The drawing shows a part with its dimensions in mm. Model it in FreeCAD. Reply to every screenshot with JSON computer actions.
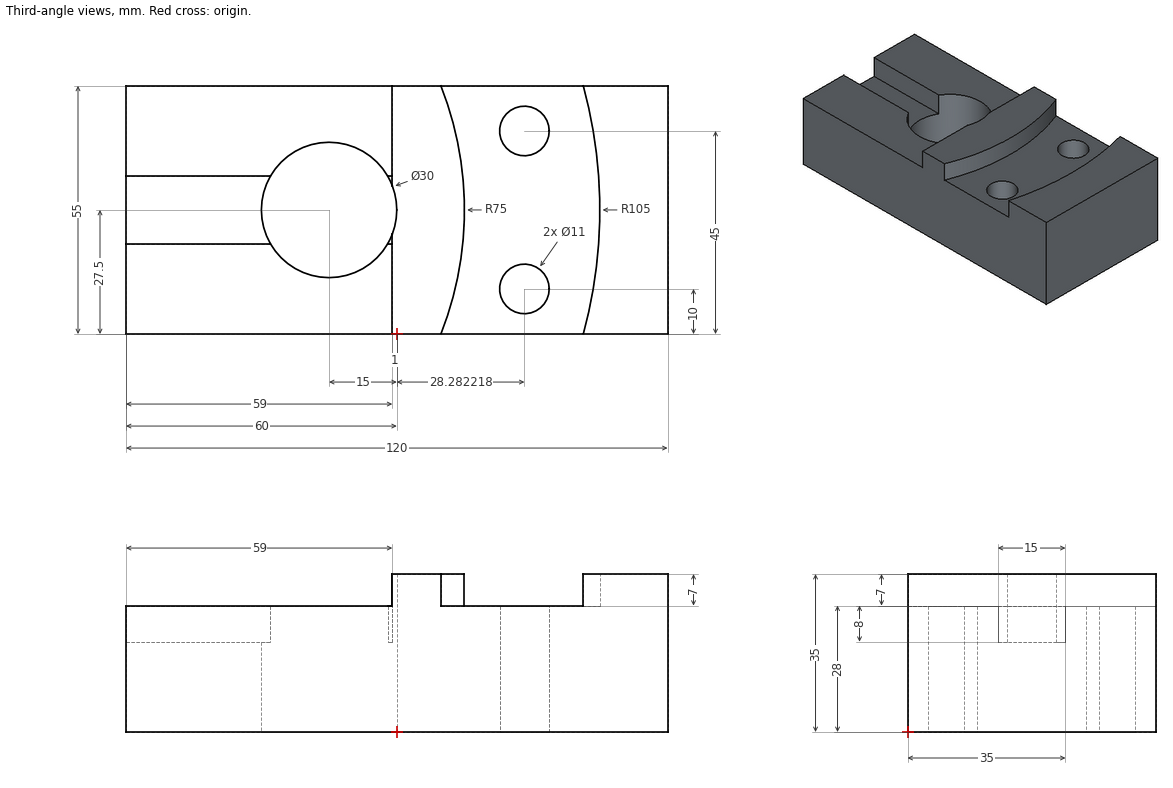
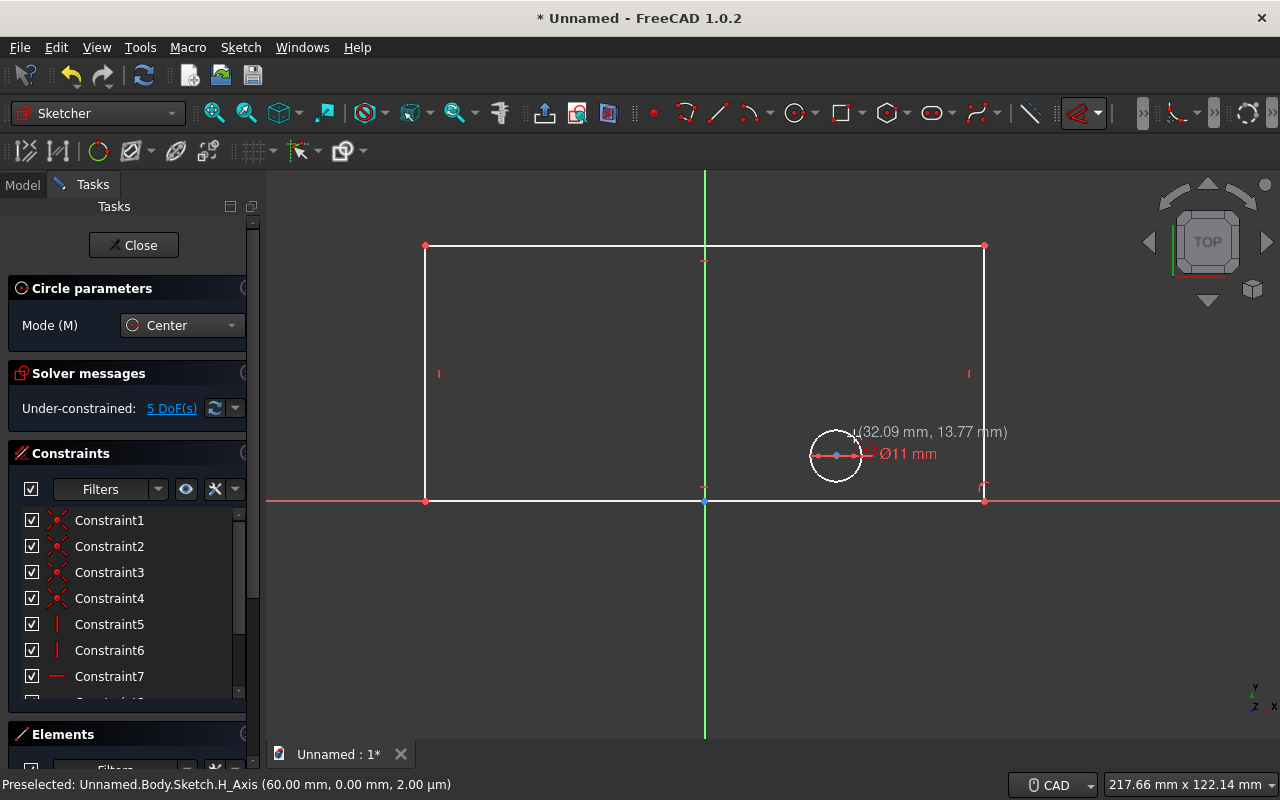
{"action": "left_click", "coordinate": [635, 373]}
{"action": "mouse_move", "coordinate": [684, 324]}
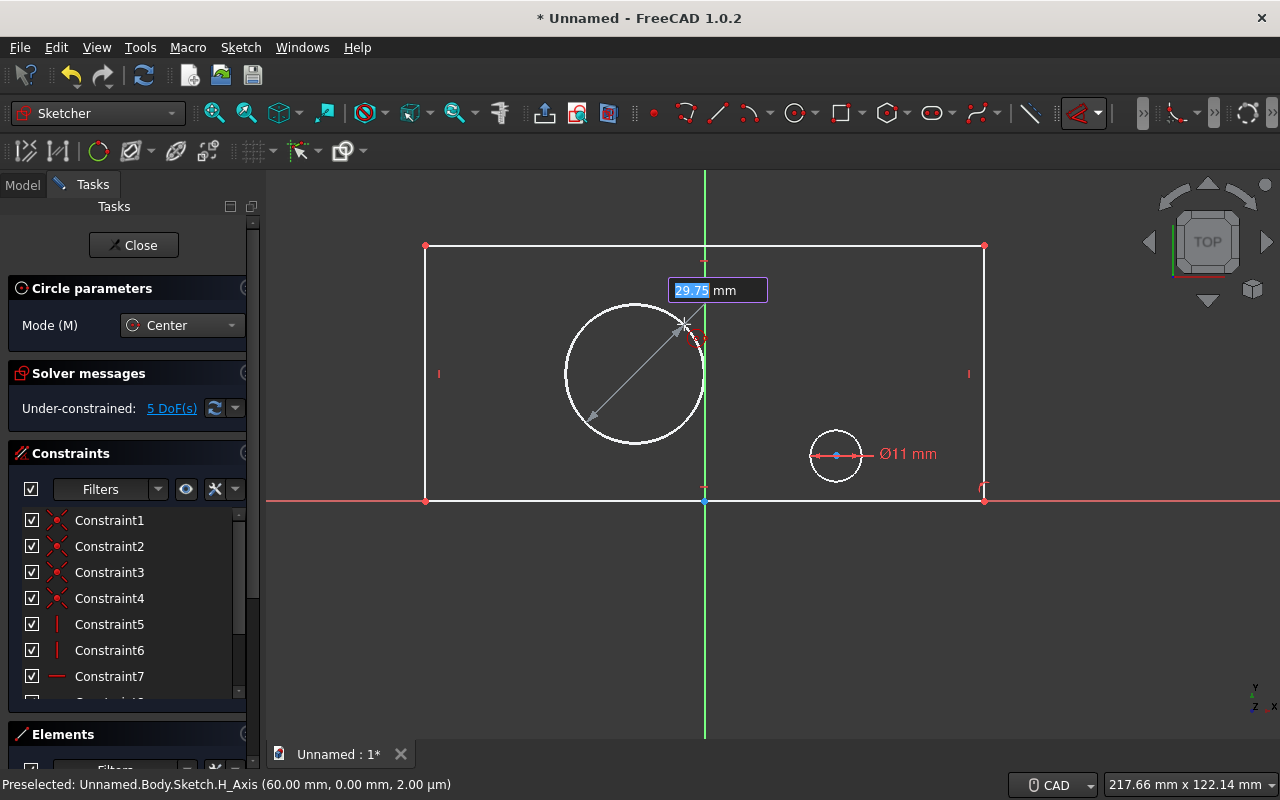
{"action": "type", "text": "30"}
{"action": "key", "text": "Return"}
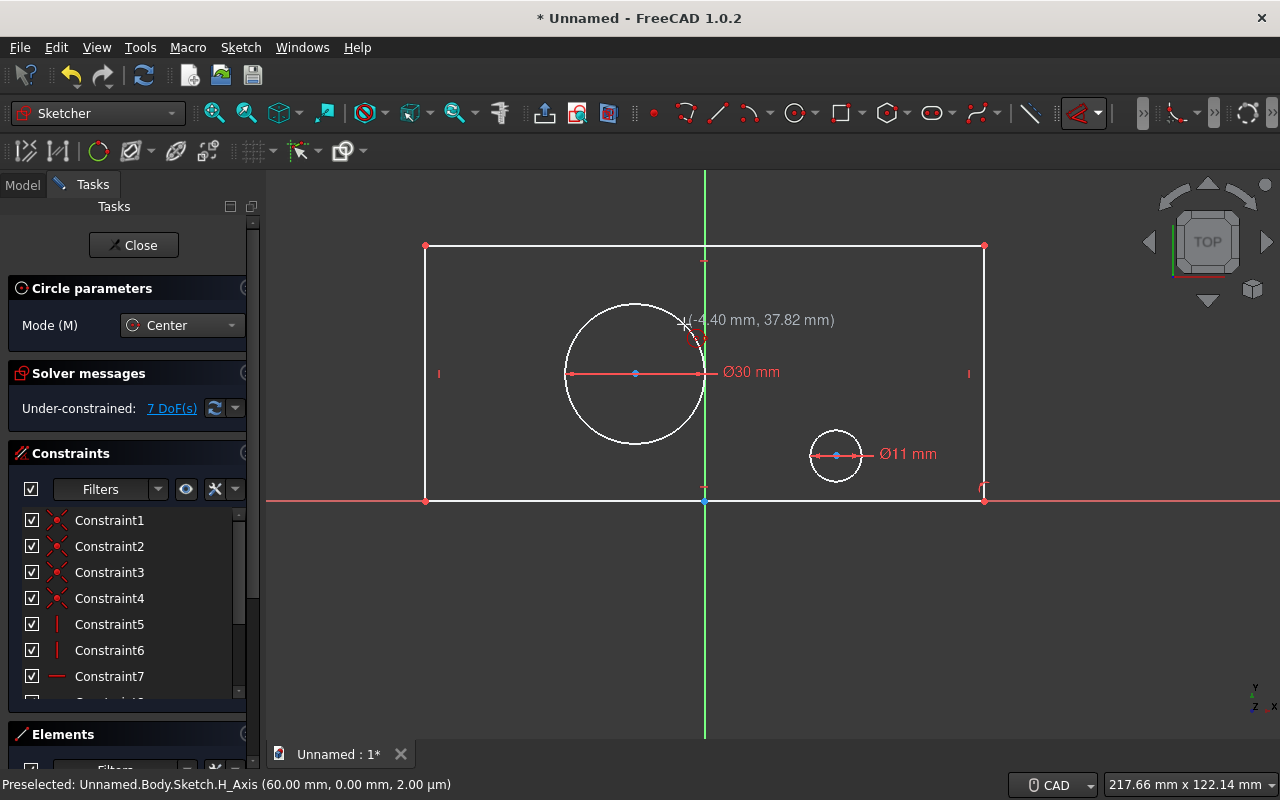
{"action": "left_click", "coordinate": [836, 292]}
{"action": "mouse_move", "coordinate": [854, 273]}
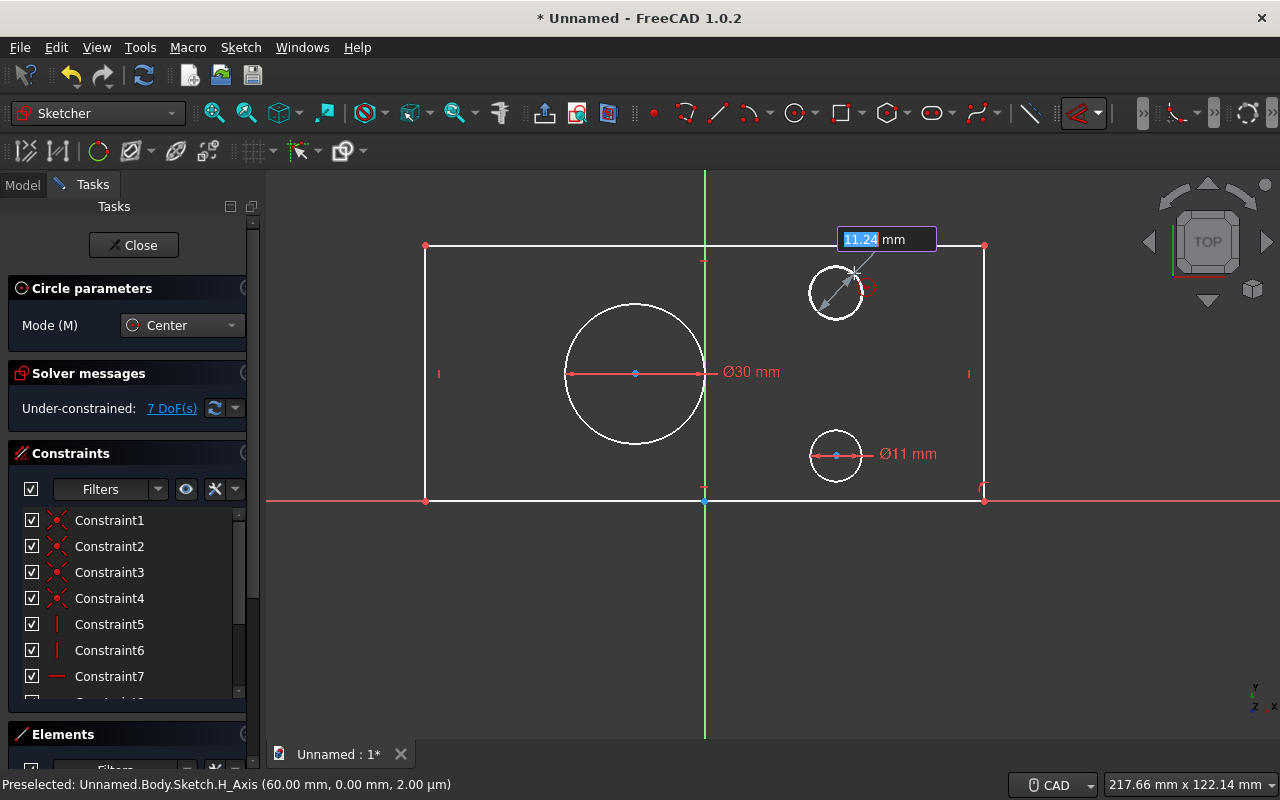
{"action": "type", "text": "11"}
{"action": "key", "text": "Return"}
{"action": "key", "text": "Escape"}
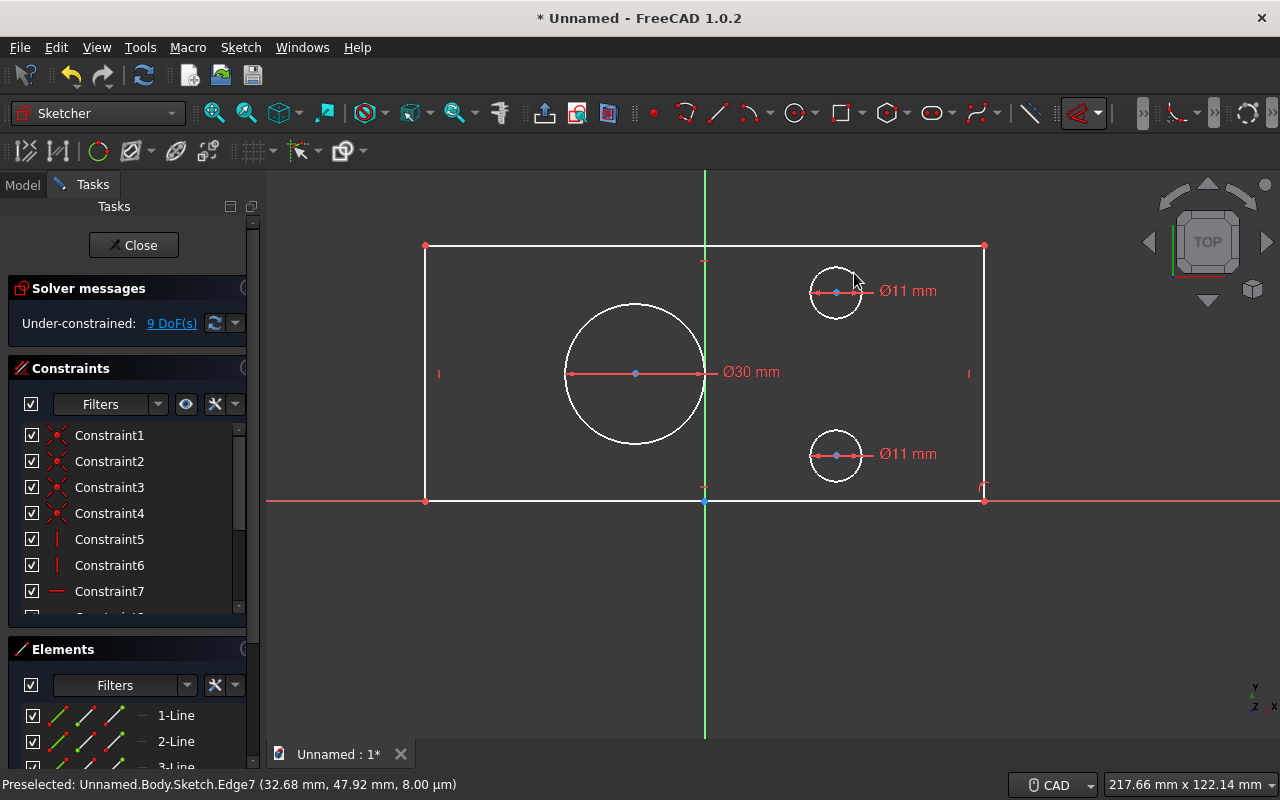
{"action": "left_click", "coordinate": [836, 456]}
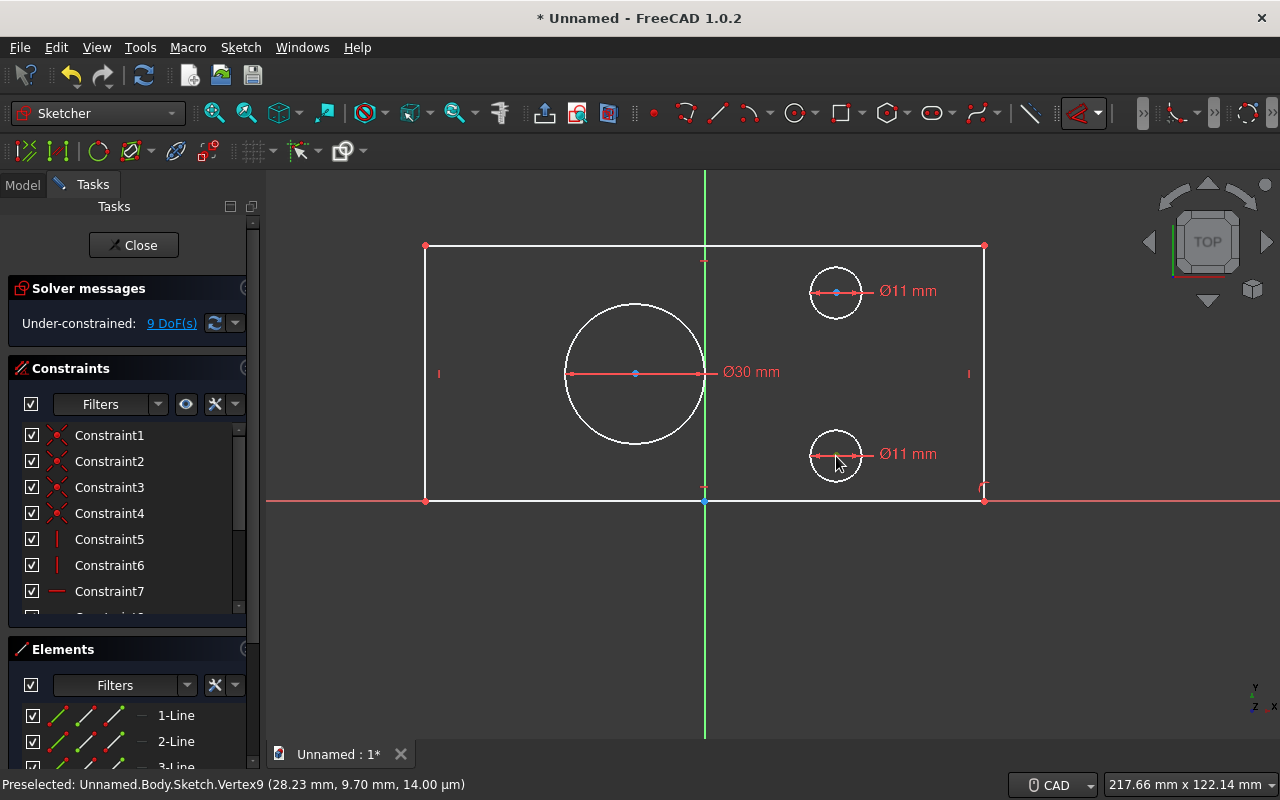
{"action": "left_click", "coordinate": [836, 293]}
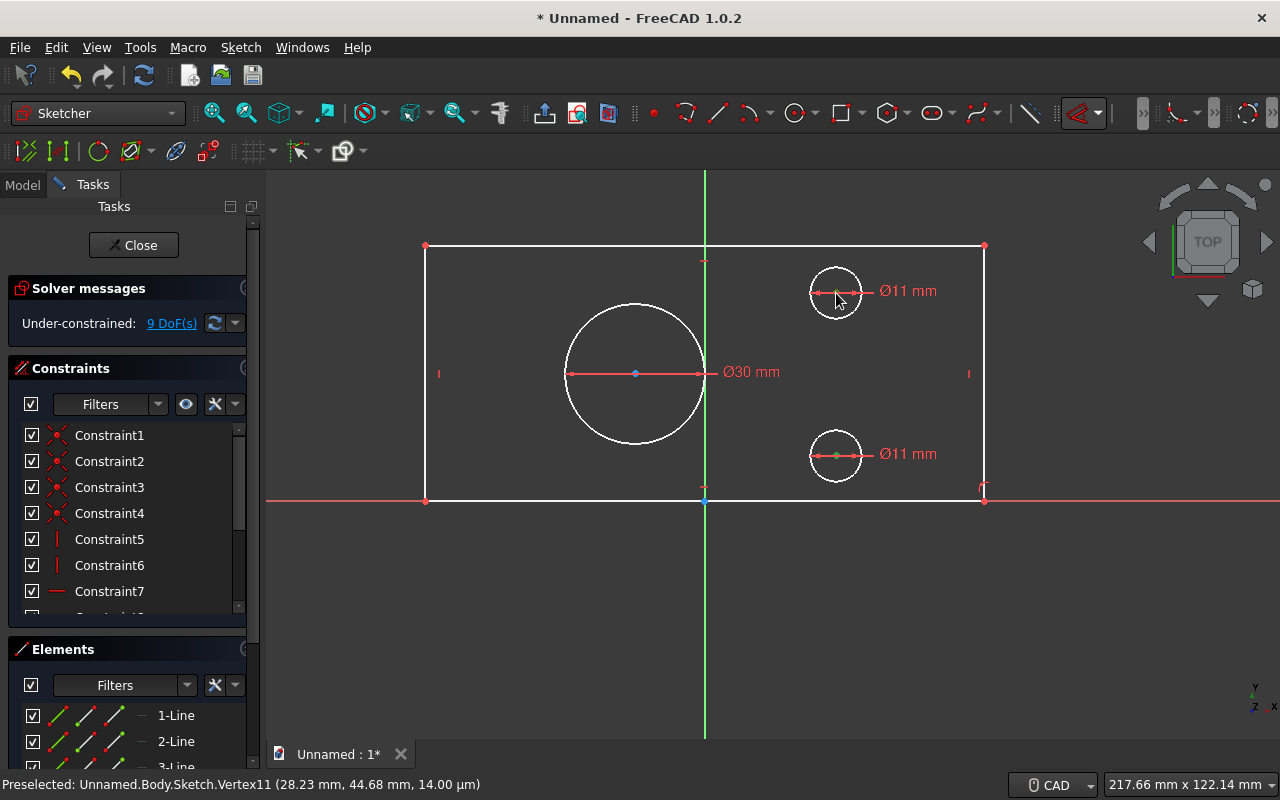
{"action": "key", "text": "v"}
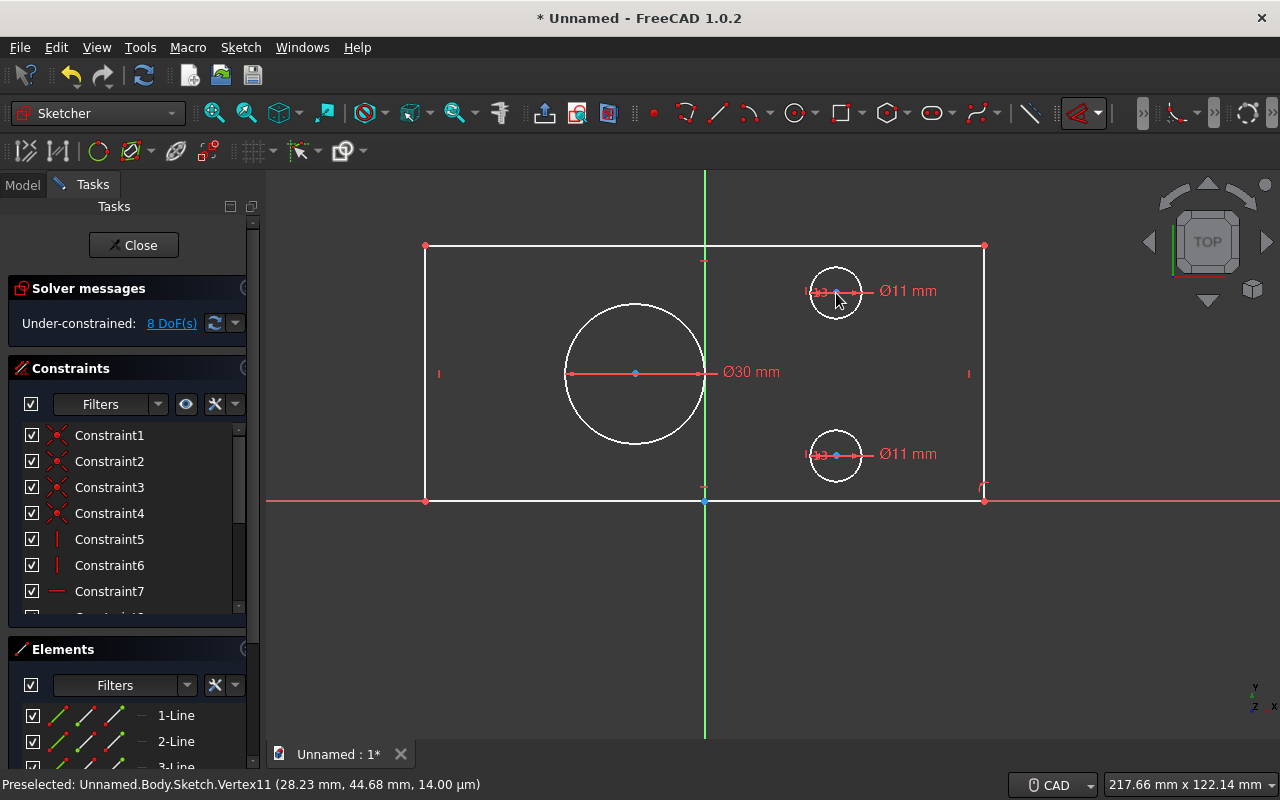
{"action": "left_click", "coordinate": [1078, 114]}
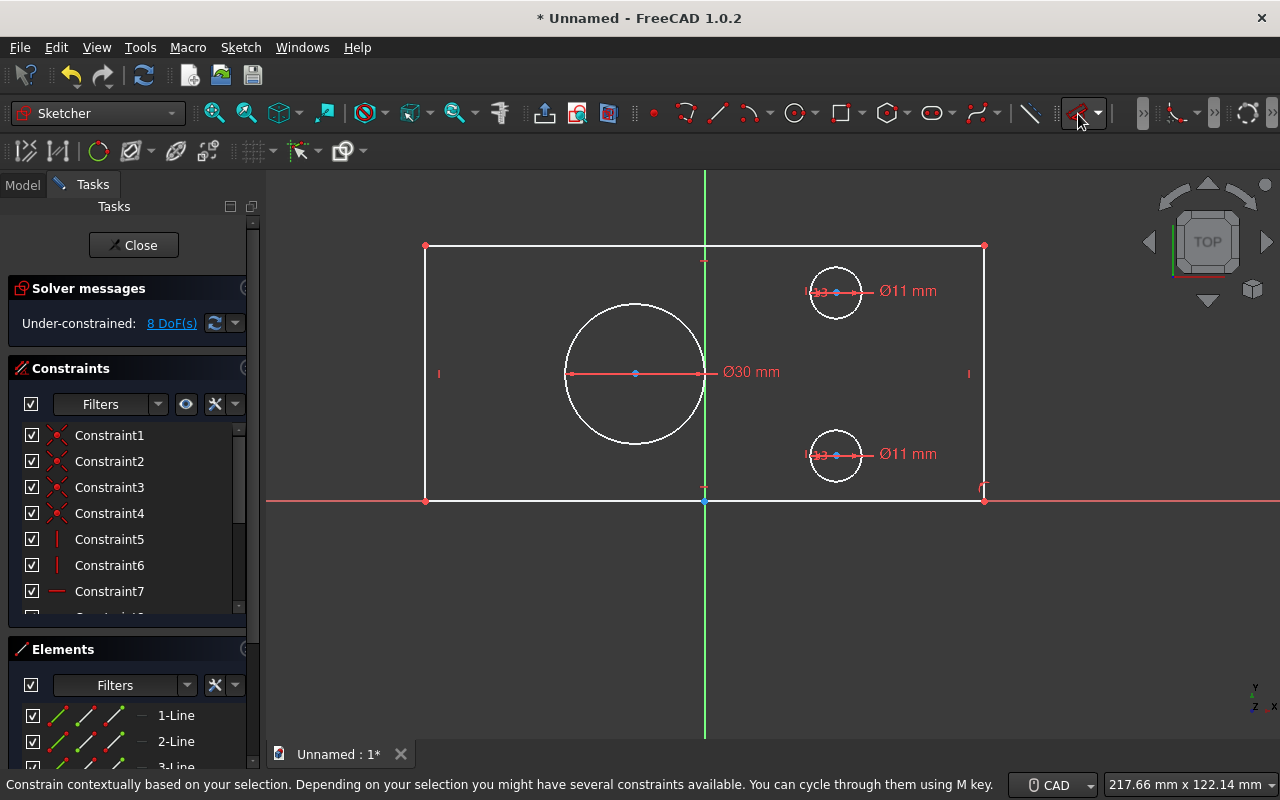
{"action": "left_click", "coordinate": [425, 323]}
{"action": "left_click", "coordinate": [391, 374]}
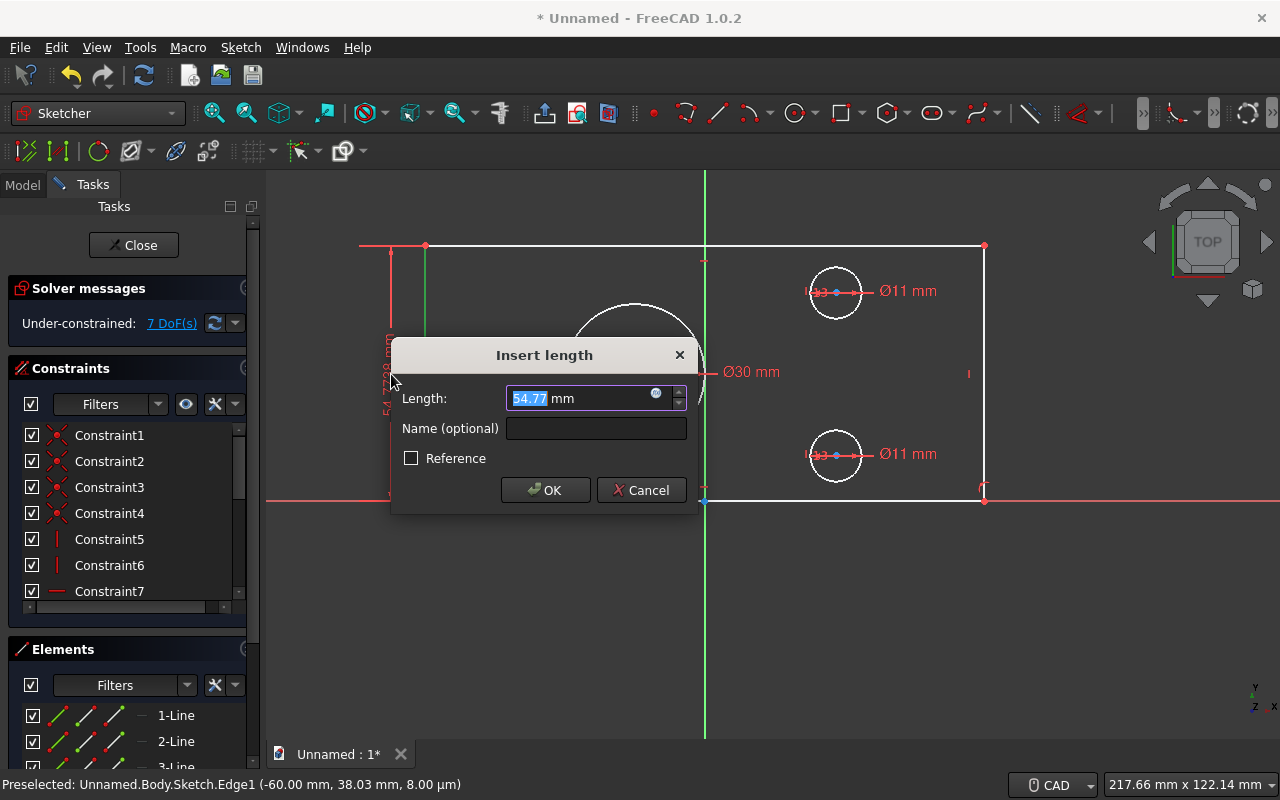
{"action": "type", "text": "55"}
{"action": "key", "text": "Return"}